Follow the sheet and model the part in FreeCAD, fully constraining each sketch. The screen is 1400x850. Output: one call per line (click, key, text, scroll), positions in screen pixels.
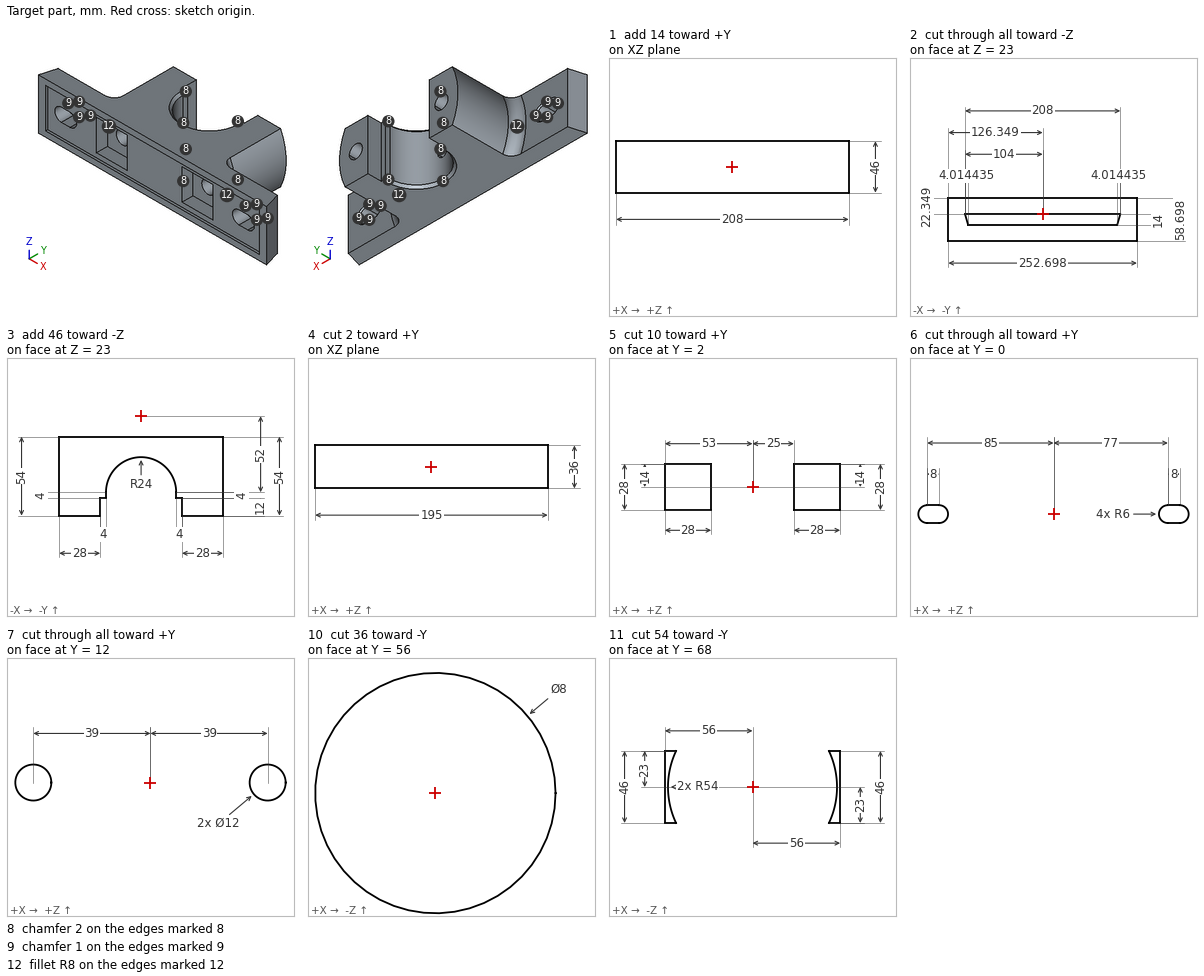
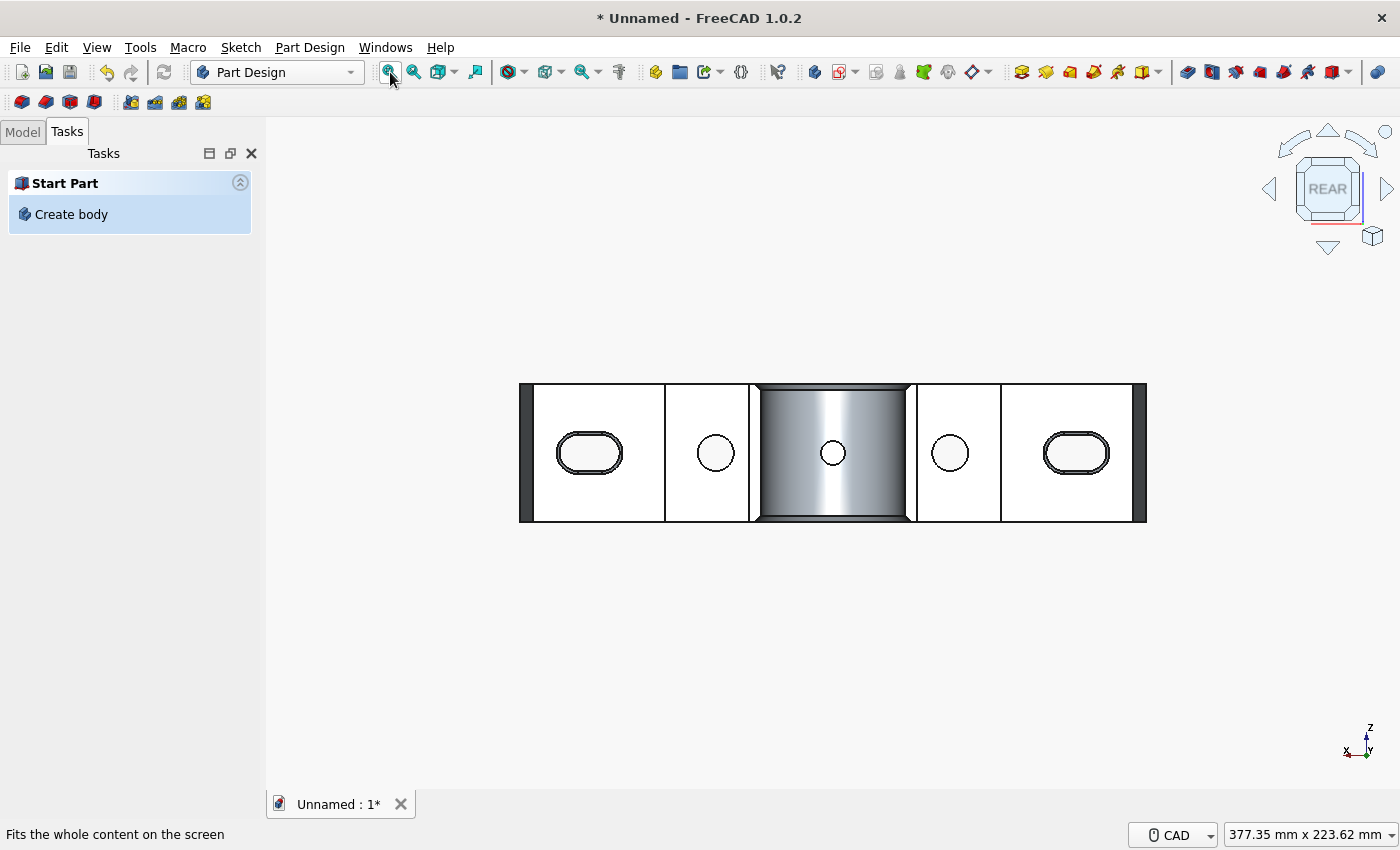
click(695, 413)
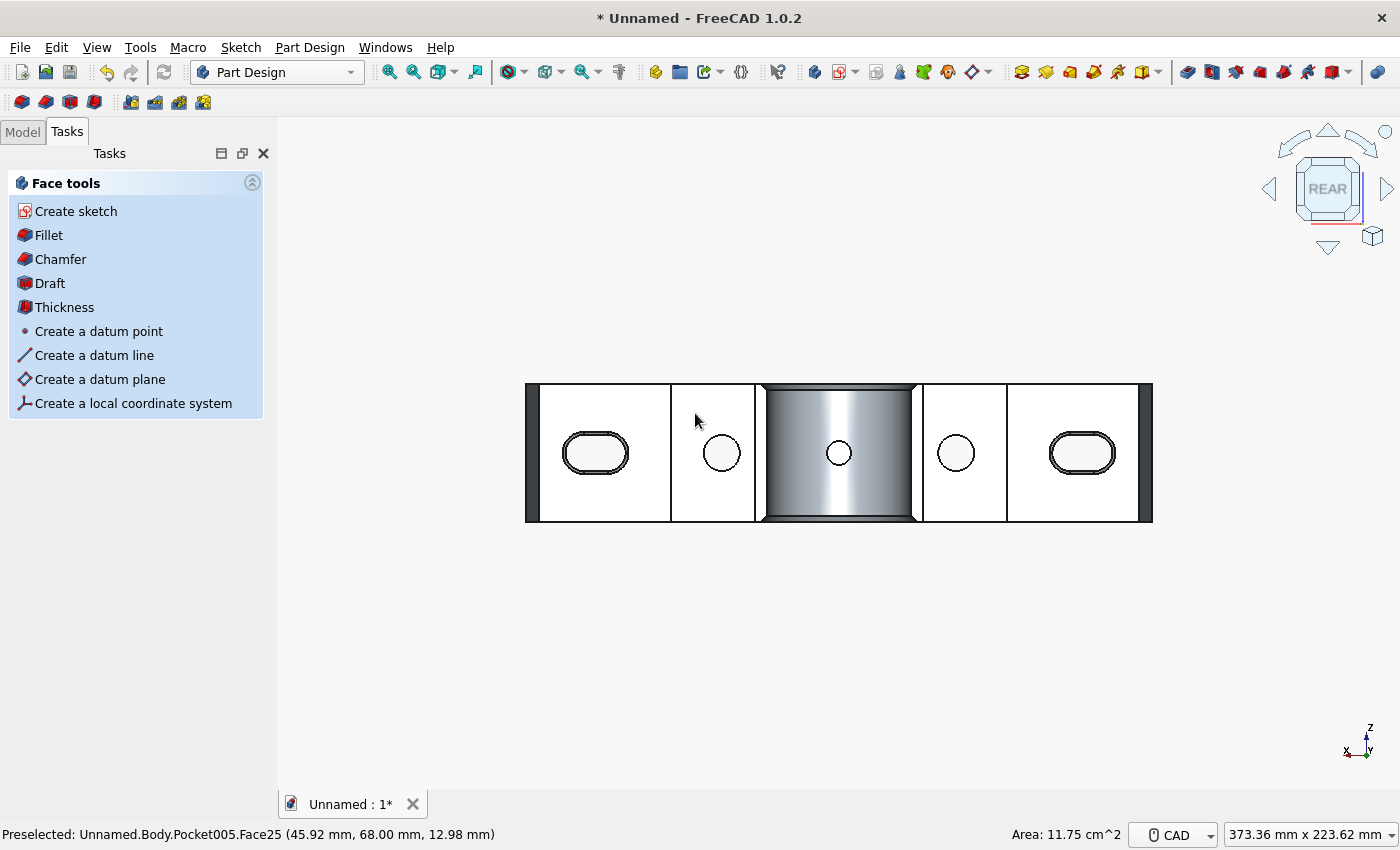
click(840, 72)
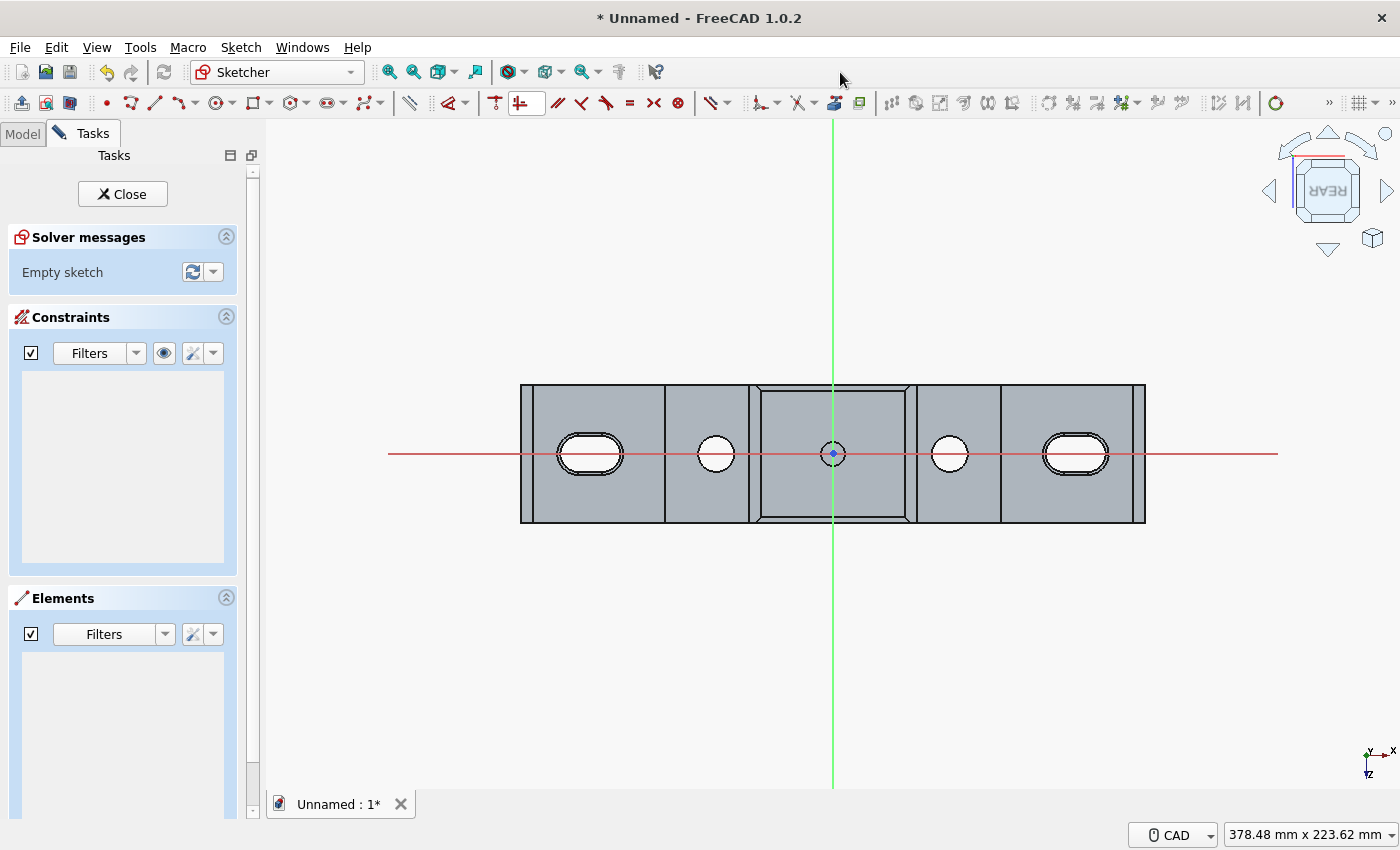
scroll(916, 454, up, 3)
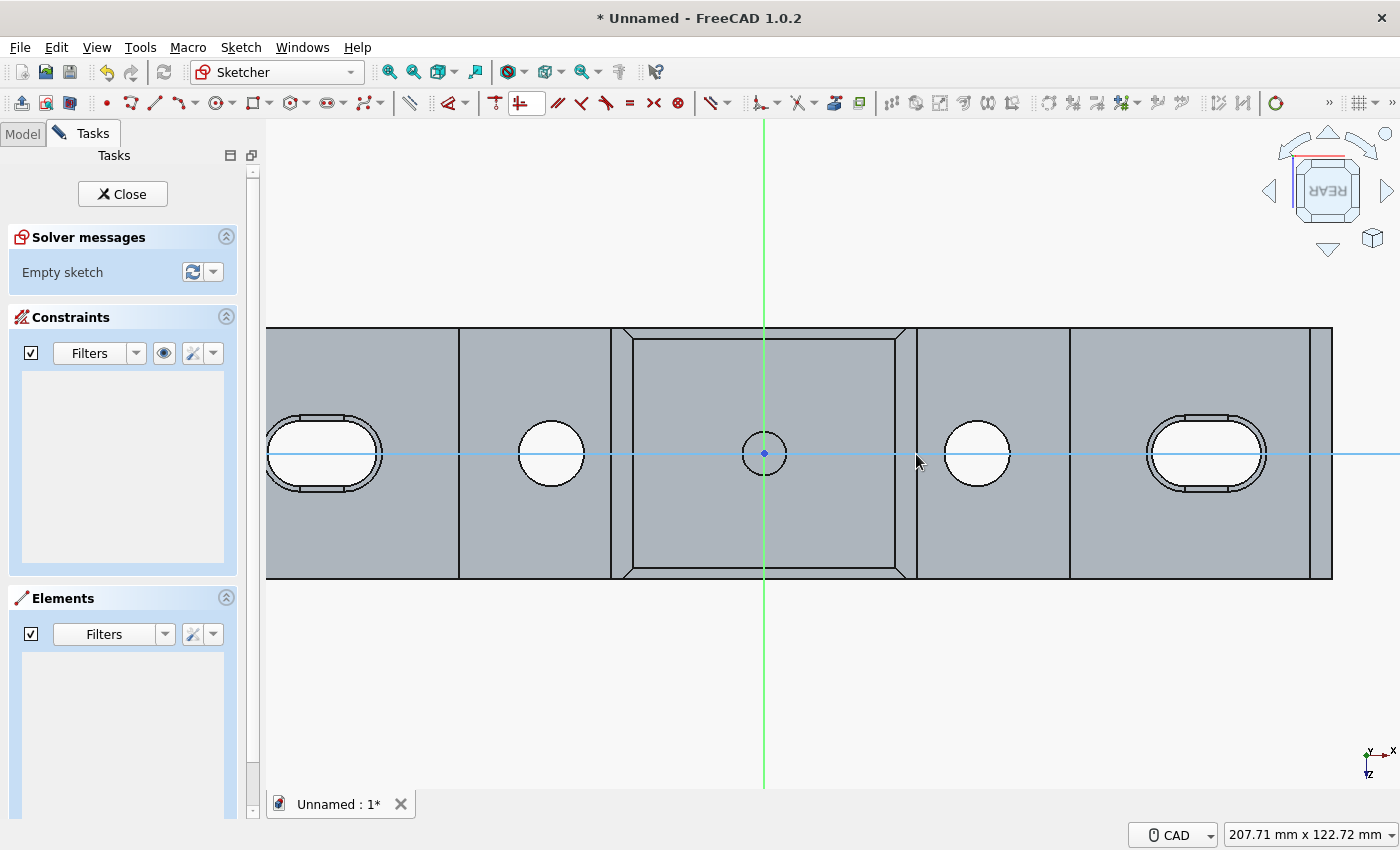
click(132, 104)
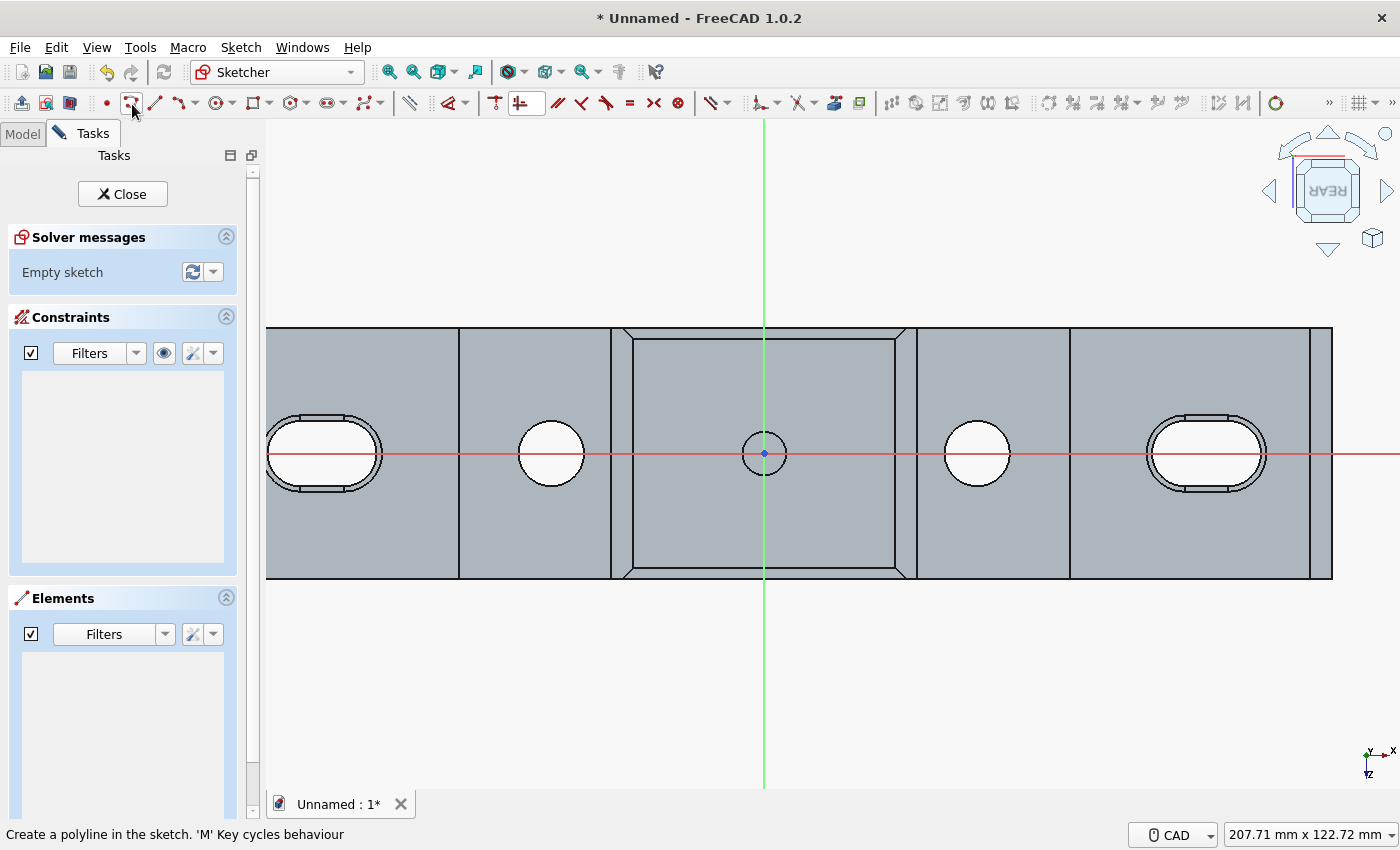
click(498, 328)
click(459, 328)
click(459, 579)
click(498, 579)
right_click(498, 579)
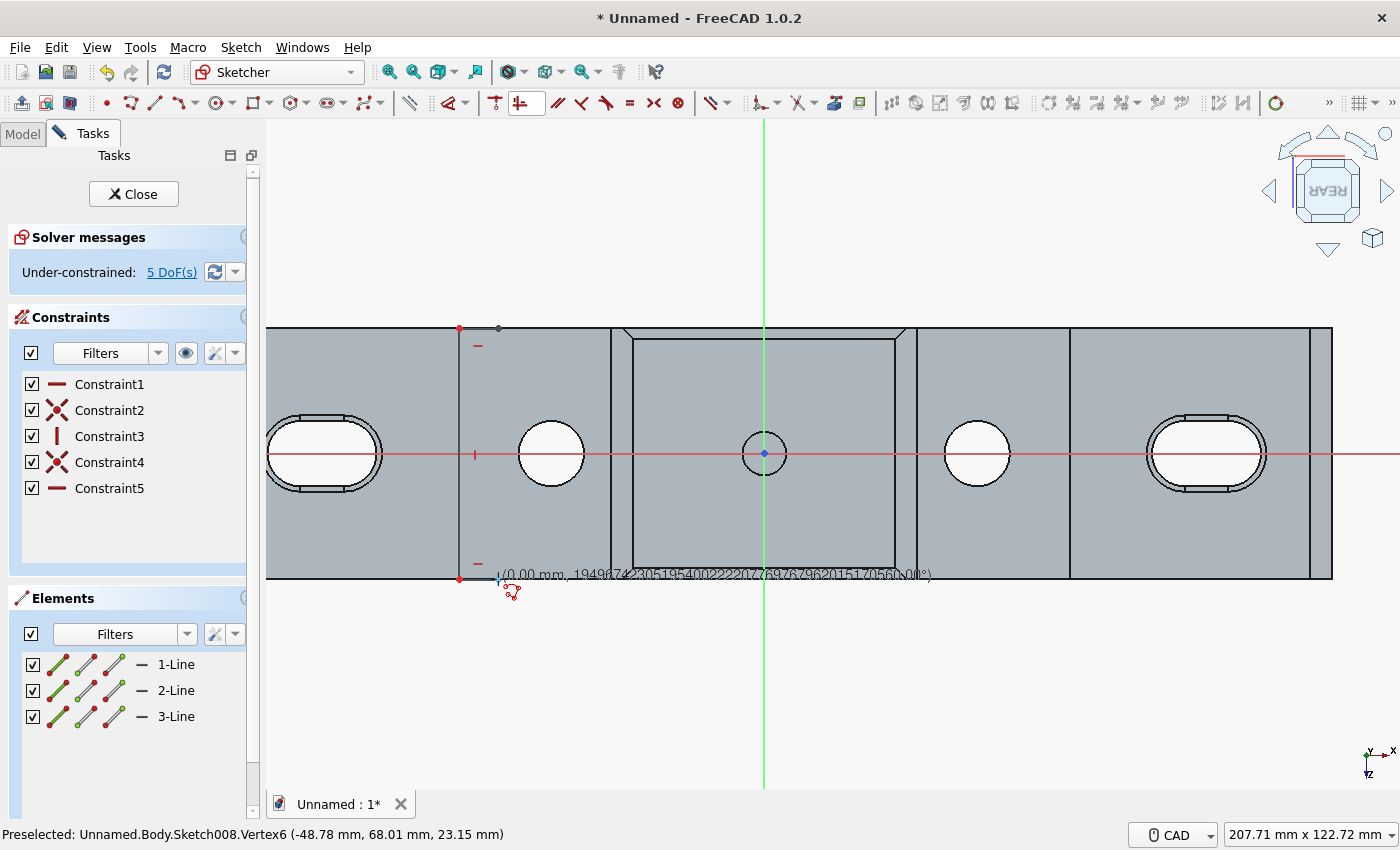
key(g)
key(3)
key(a)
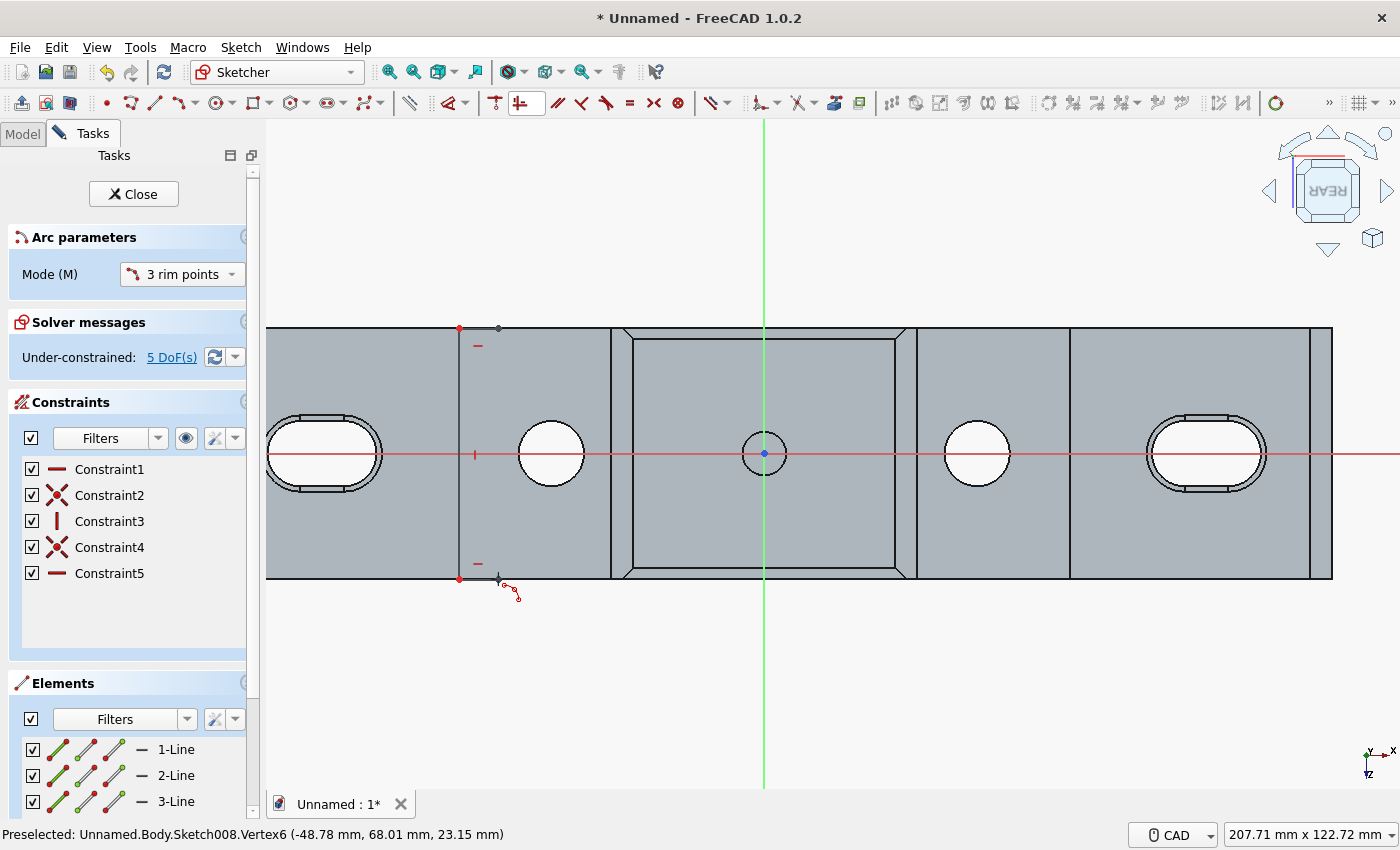
click(498, 580)
click(498, 329)
click(474, 402)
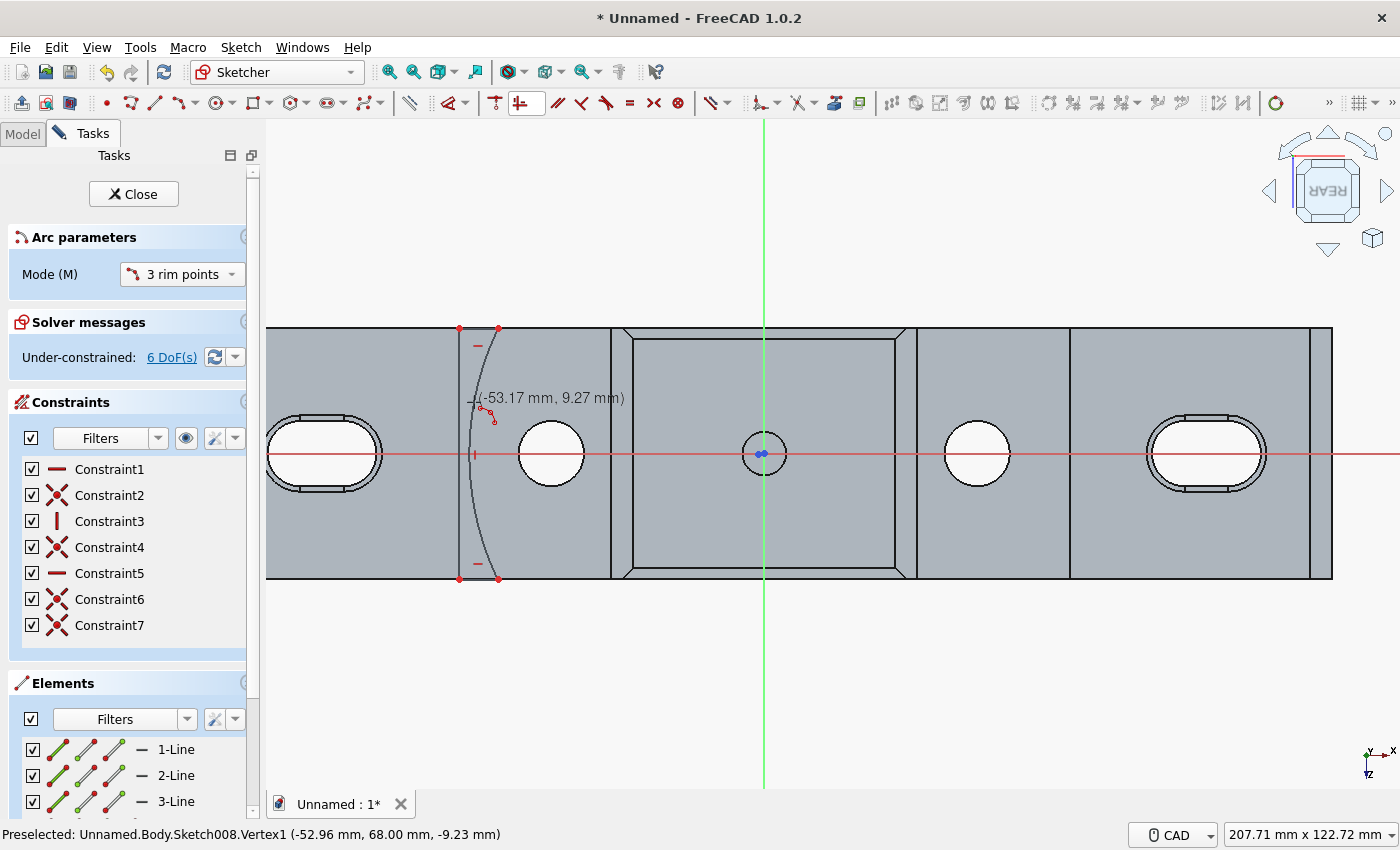
click(132, 104)